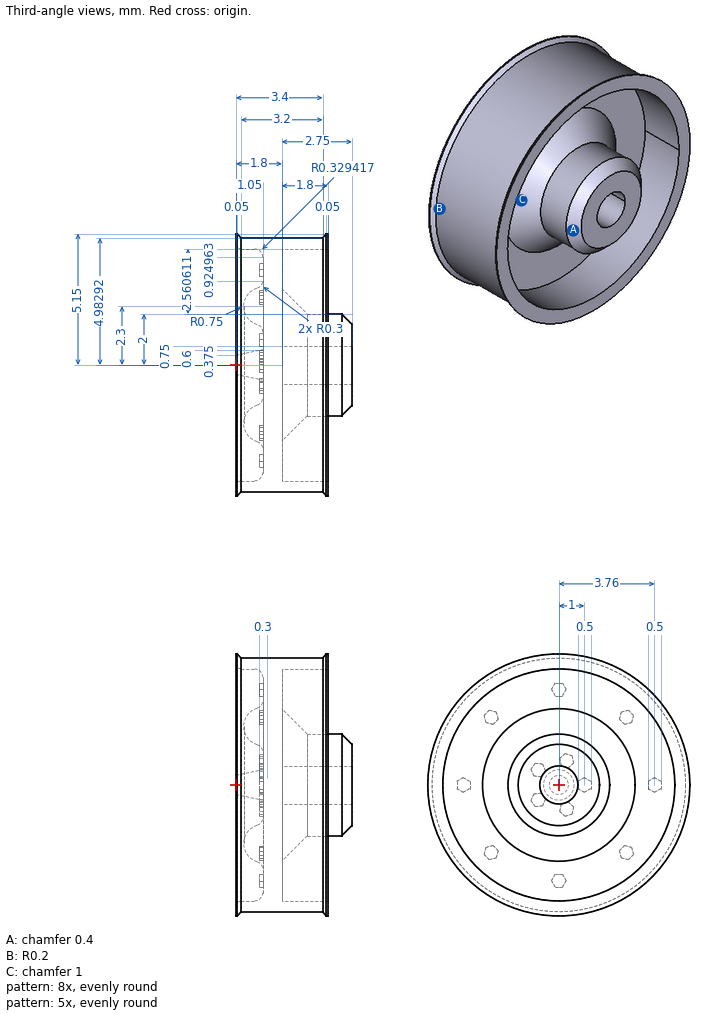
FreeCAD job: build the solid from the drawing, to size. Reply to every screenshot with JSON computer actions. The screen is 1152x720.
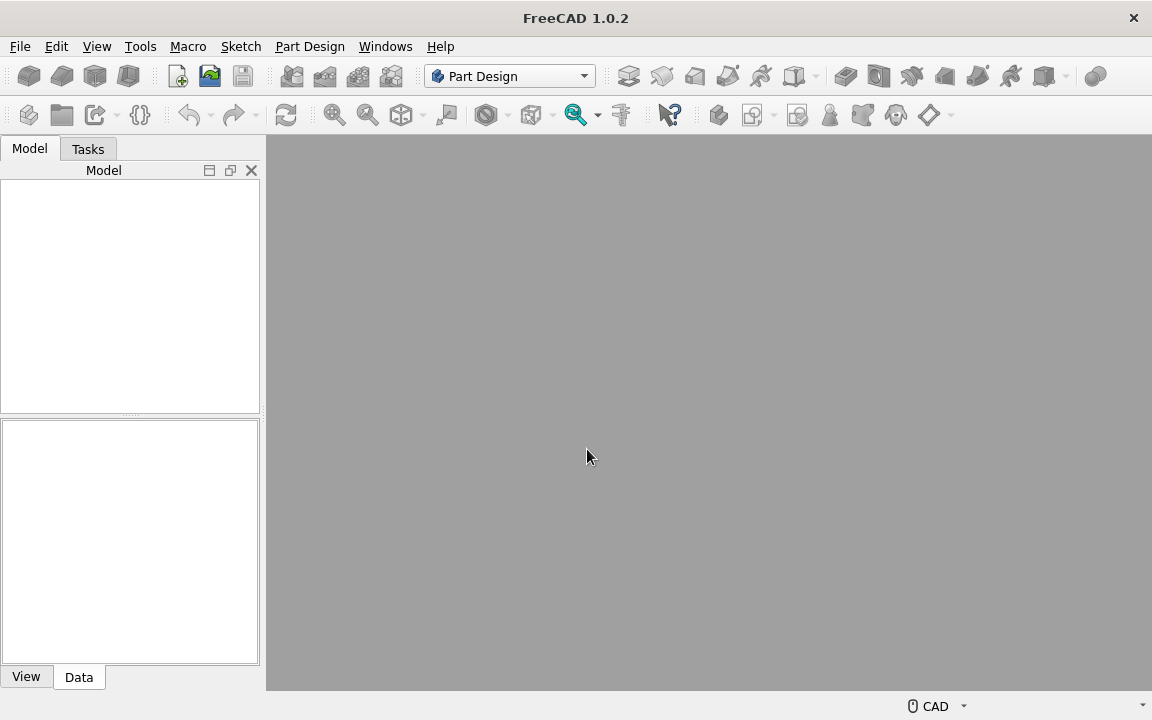
{"action": "left_click", "coordinate": [177, 76]}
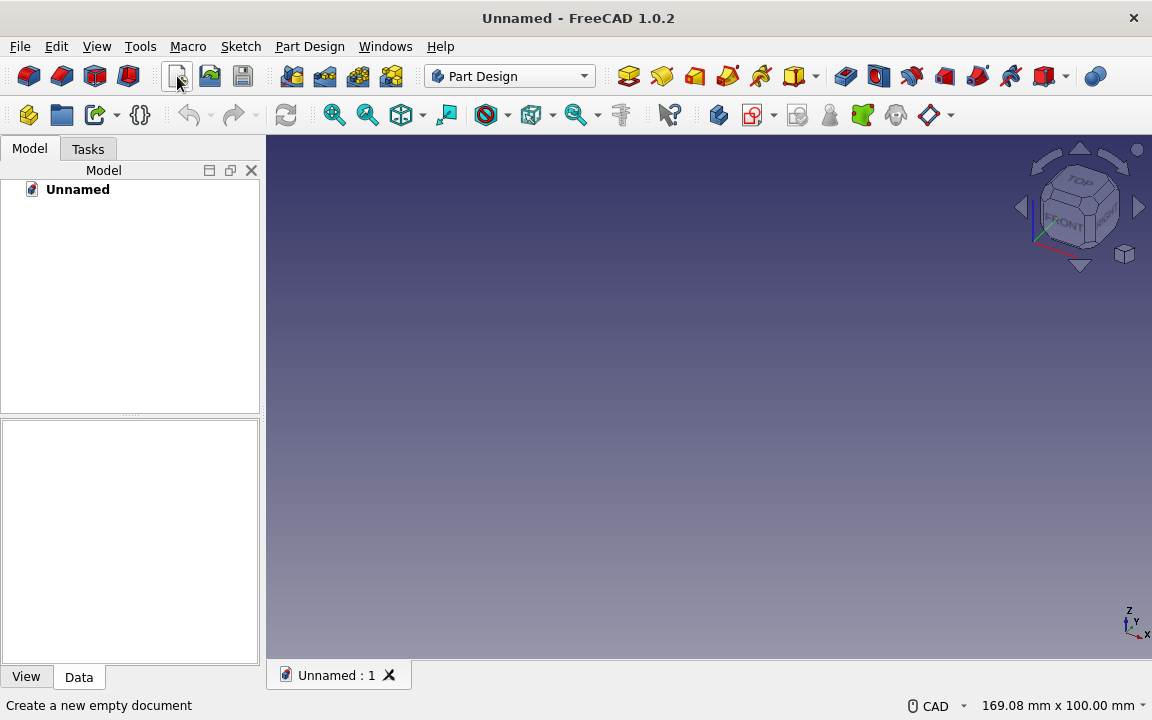
{"action": "left_click", "coordinate": [752, 116]}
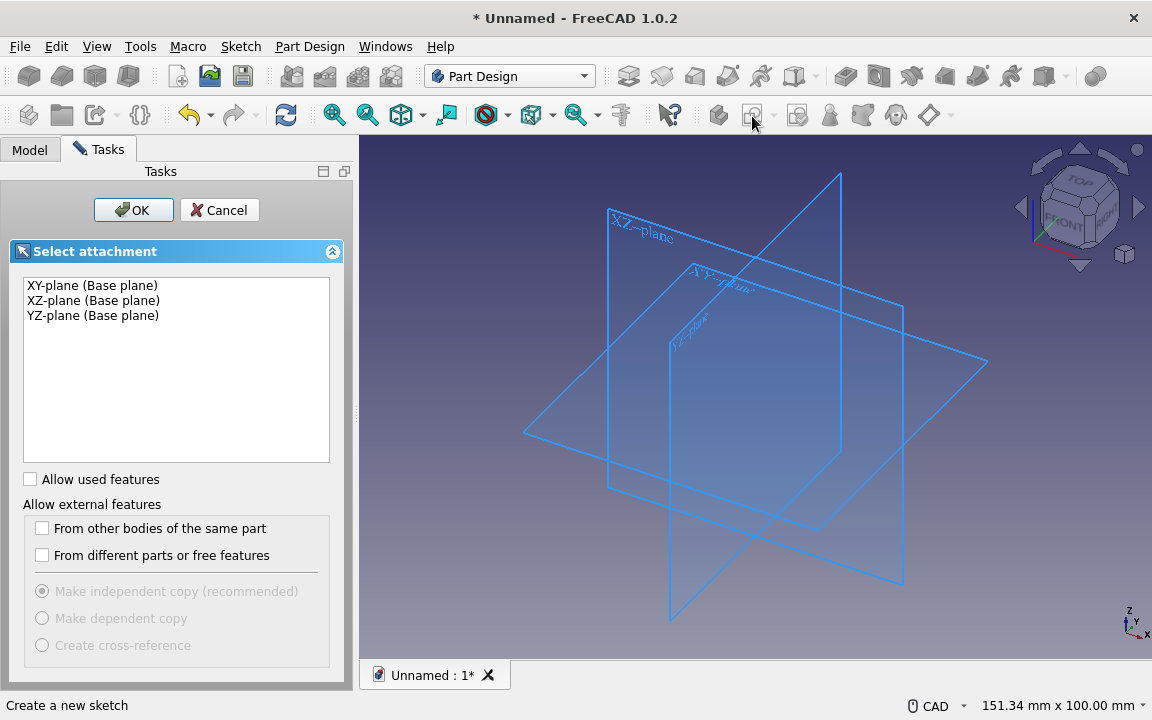
{"action": "left_click", "coordinate": [84, 286]}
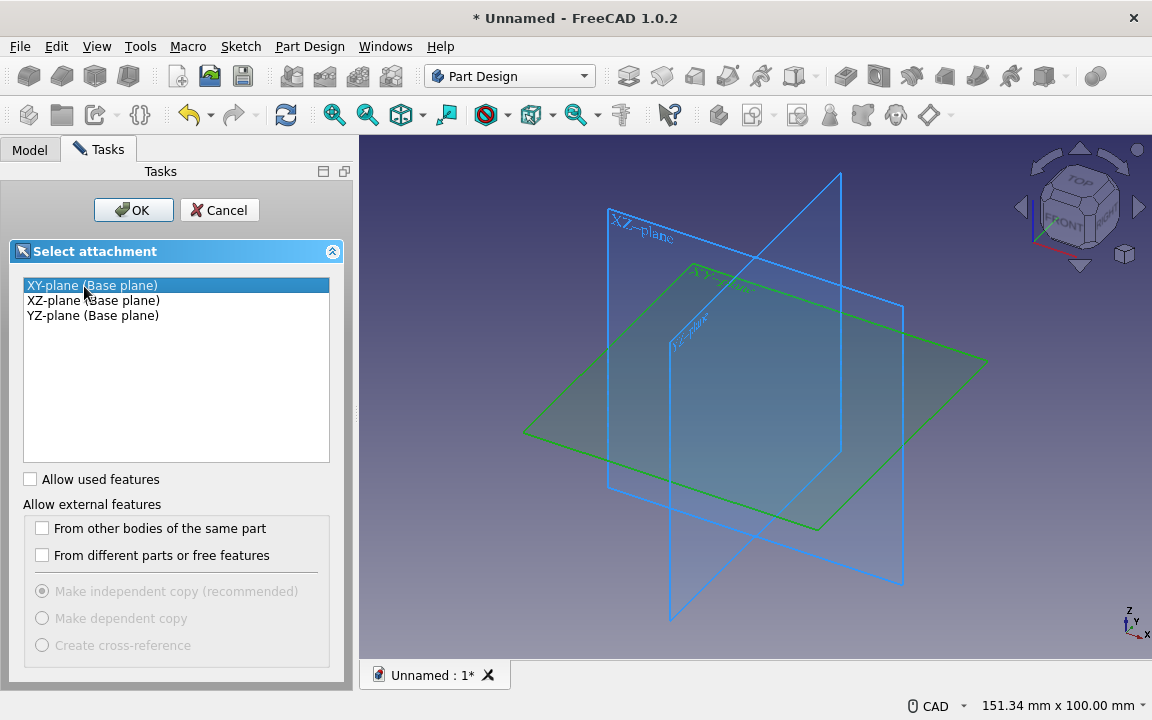
{"action": "left_click", "coordinate": [134, 210]}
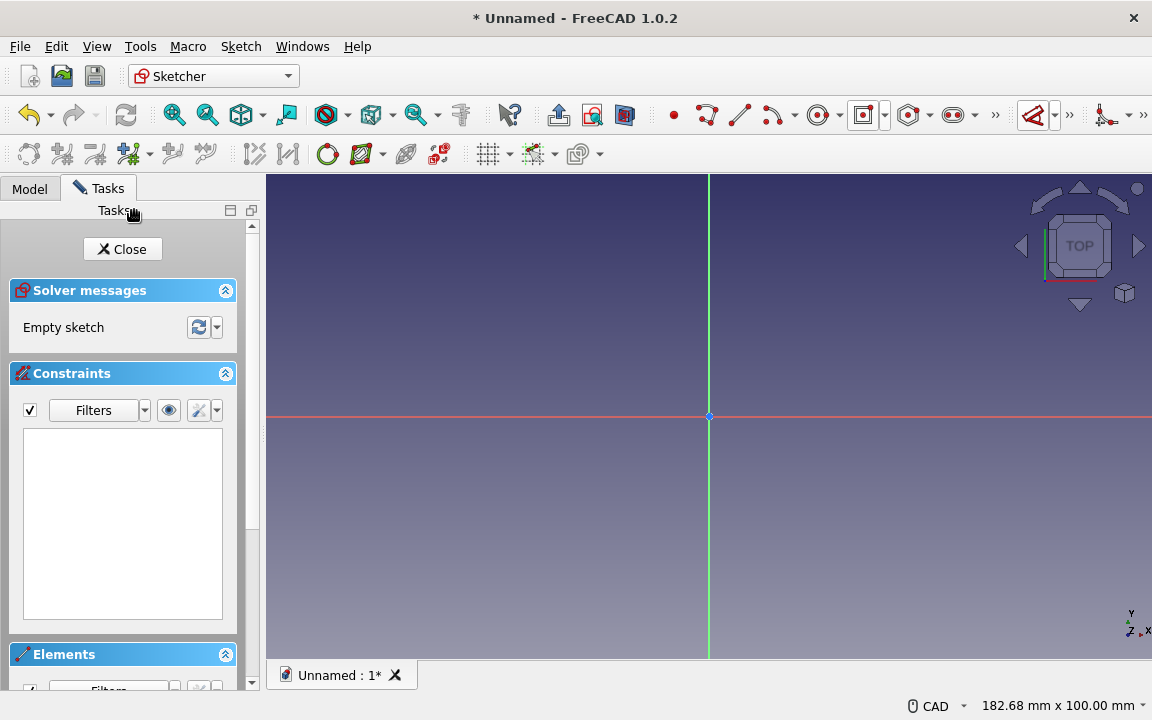
{"action": "scroll", "coordinate": [728, 403], "scroll_direction": "up", "scroll_amount": 12}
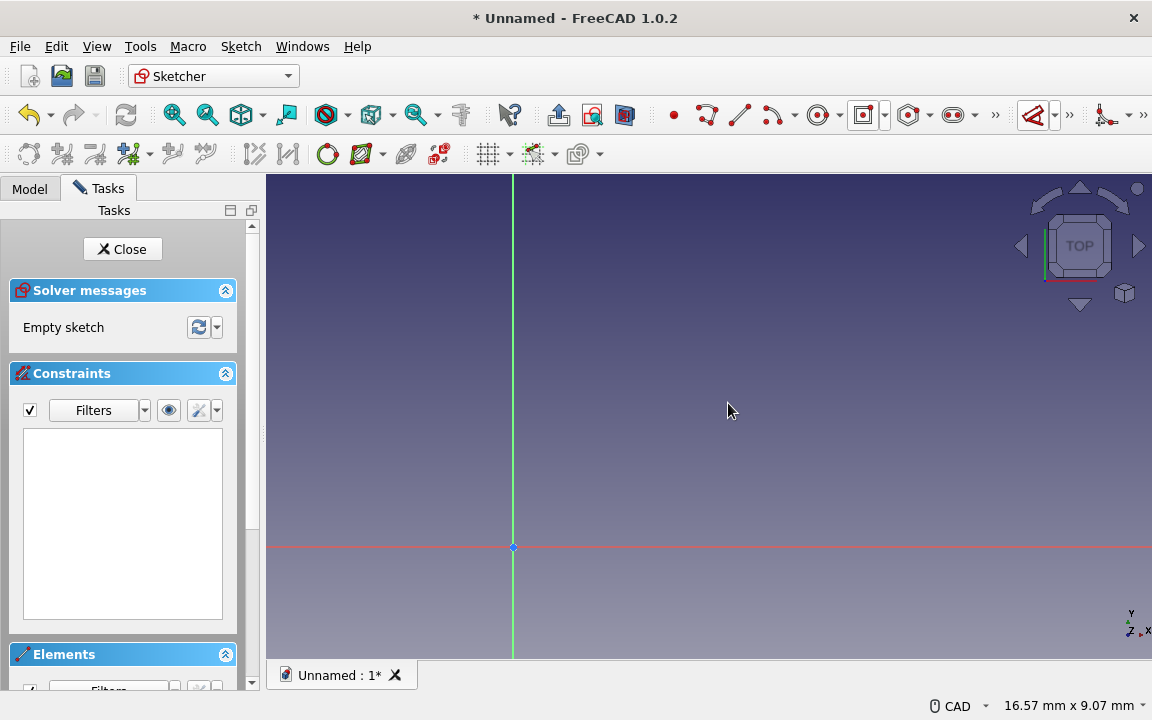
{"action": "left_click", "coordinate": [740, 116]}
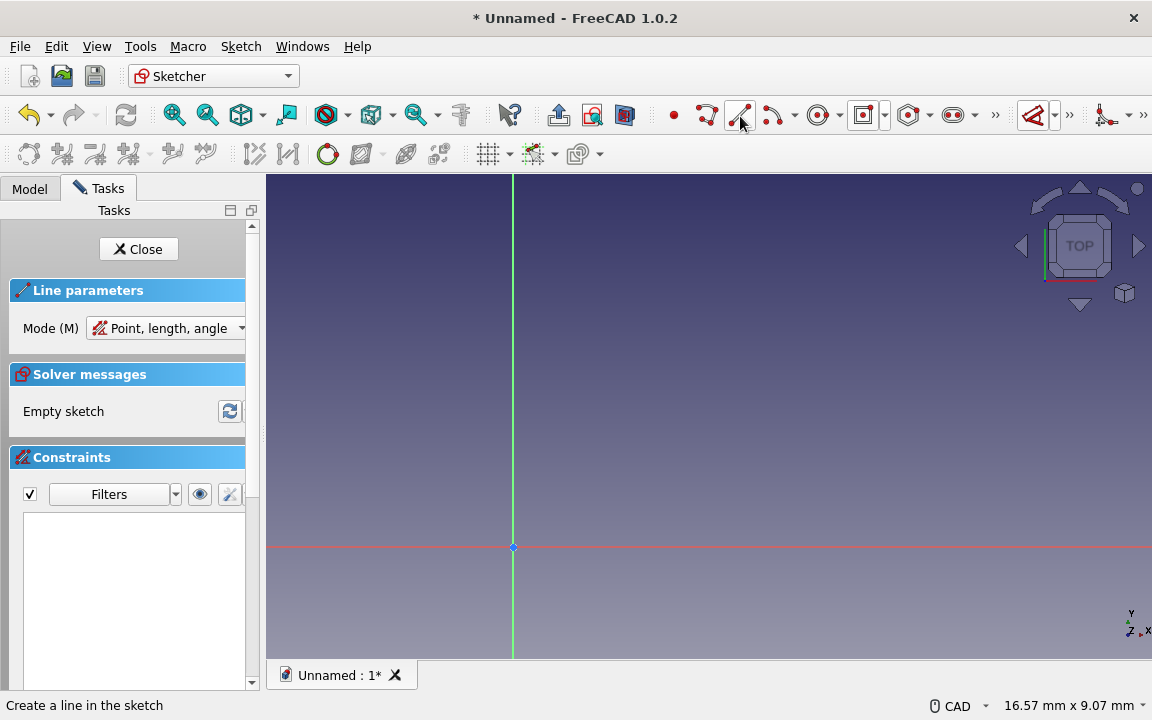
{"action": "left_click", "coordinate": [569, 321]}
{"action": "left_click", "coordinate": [569, 370]}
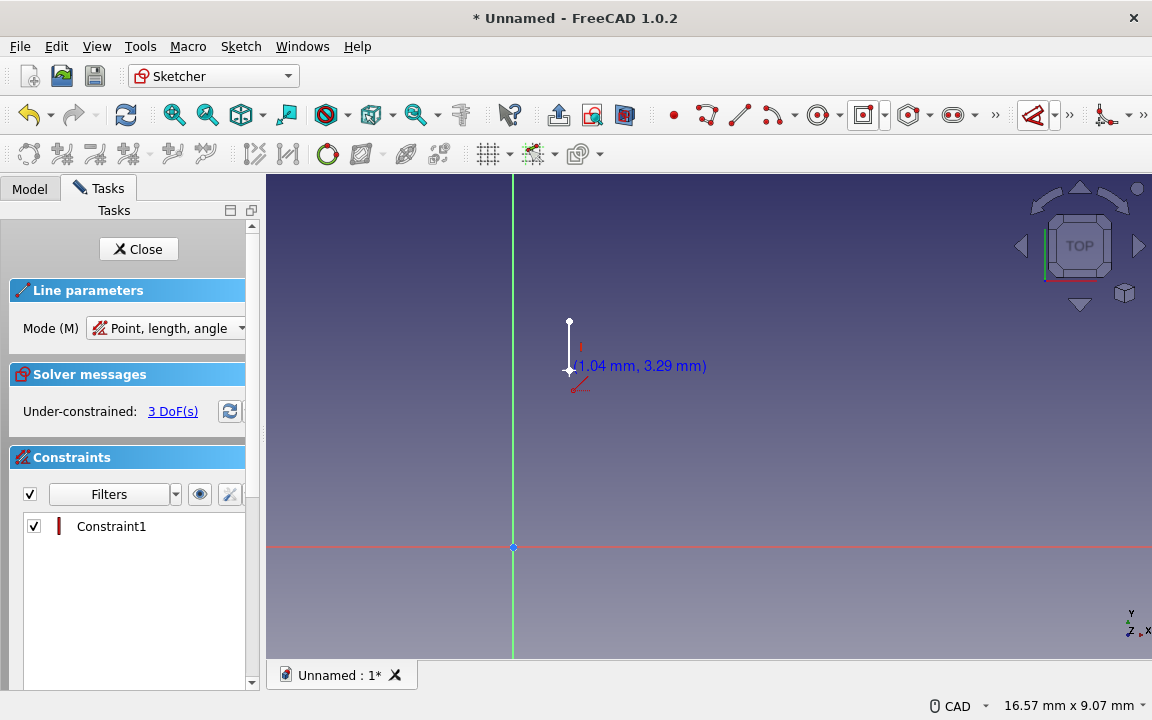
{"action": "left_click", "coordinate": [707, 116]}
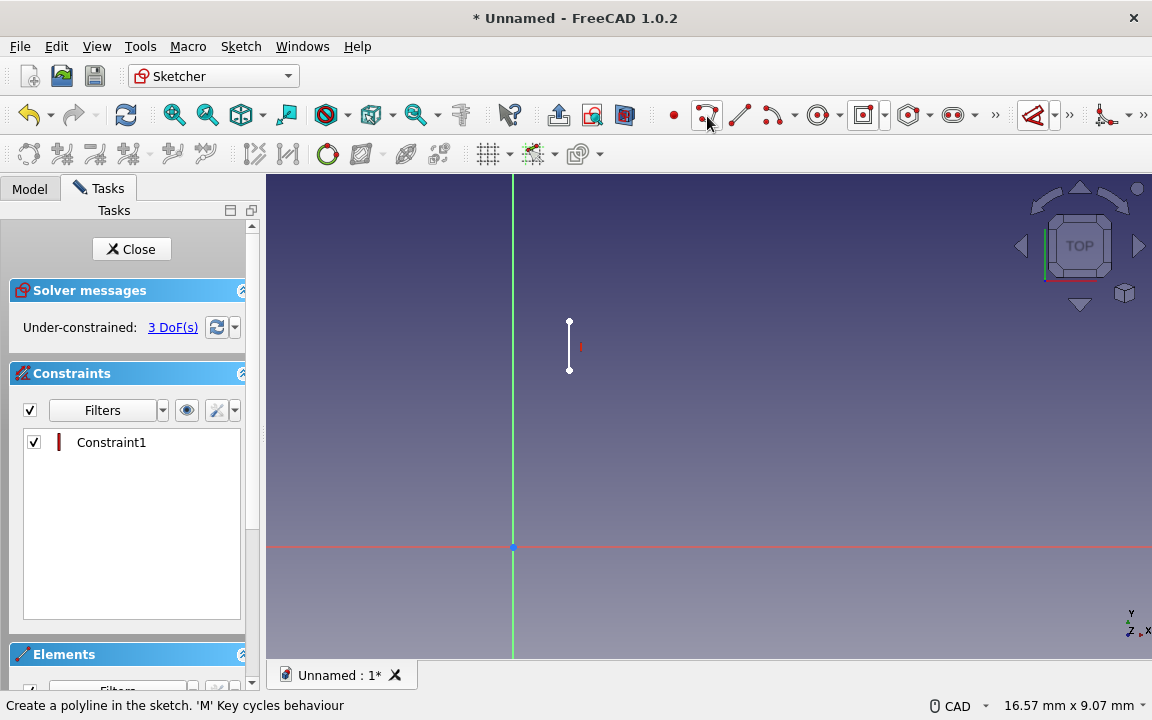
{"action": "left_click", "coordinate": [569, 478]}
{"action": "left_click", "coordinate": [569, 515]}
{"action": "left_click", "coordinate": [513, 527]}
{"action": "left_click", "coordinate": [513, 547]}
{"action": "left_click", "coordinate": [610, 538]}
{"action": "left_click", "coordinate": [610, 507]}
{"action": "left_click", "coordinate": [757, 507]}
{"action": "left_click", "coordinate": [757, 440]}
{"action": "left_click", "coordinate": [610, 440]}
{"action": "left_click", "coordinate": [610, 303]}
{"action": "left_click", "coordinate": [706, 303]}
{"action": "left_click", "coordinate": [706, 272]}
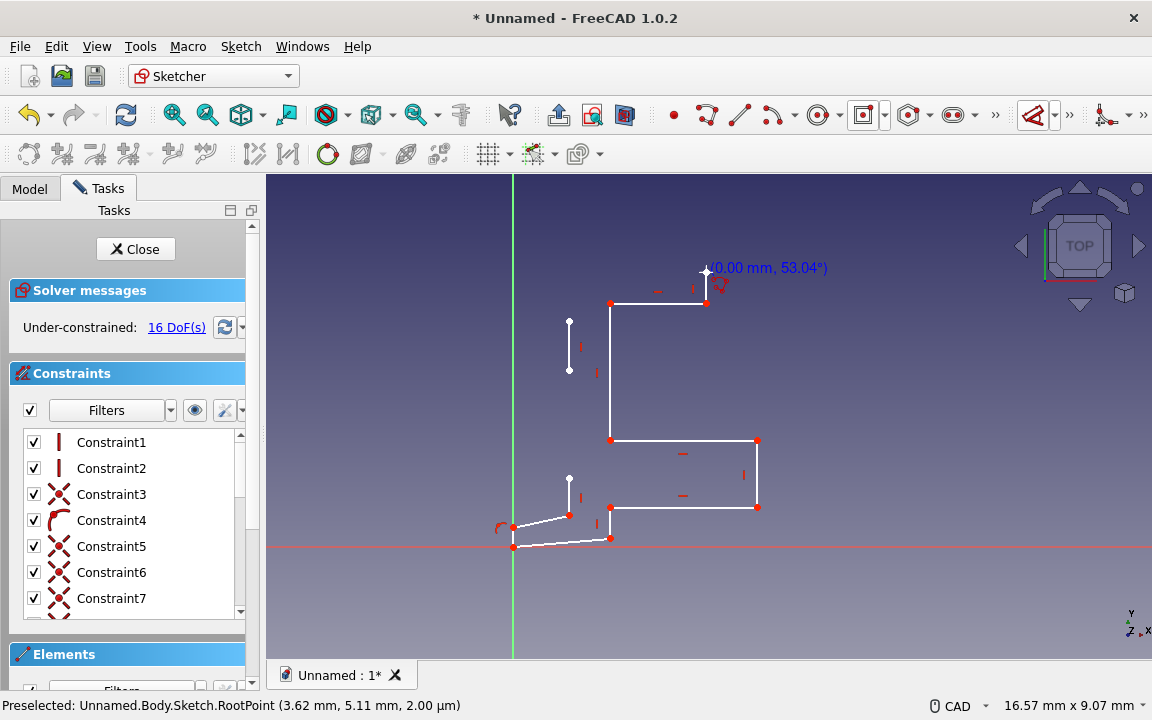
{"action": "scroll", "coordinate": [703, 272], "scroll_direction": "up", "scroll_amount": 9}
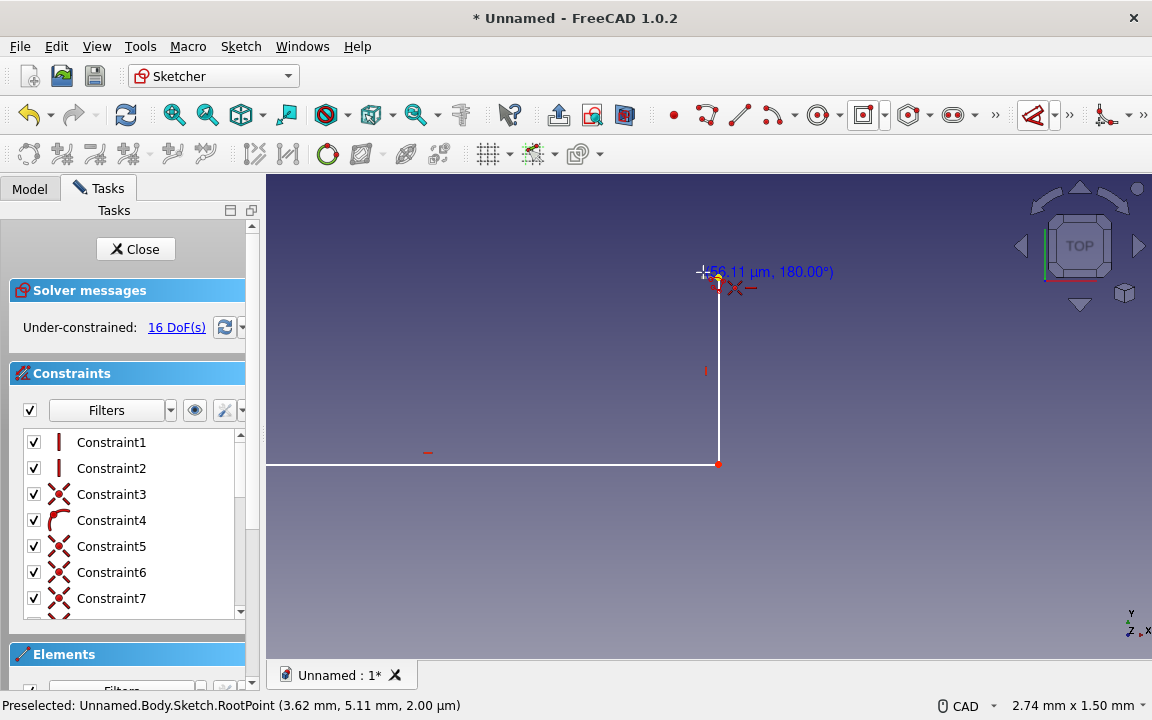
{"action": "left_click", "coordinate": [701, 271]}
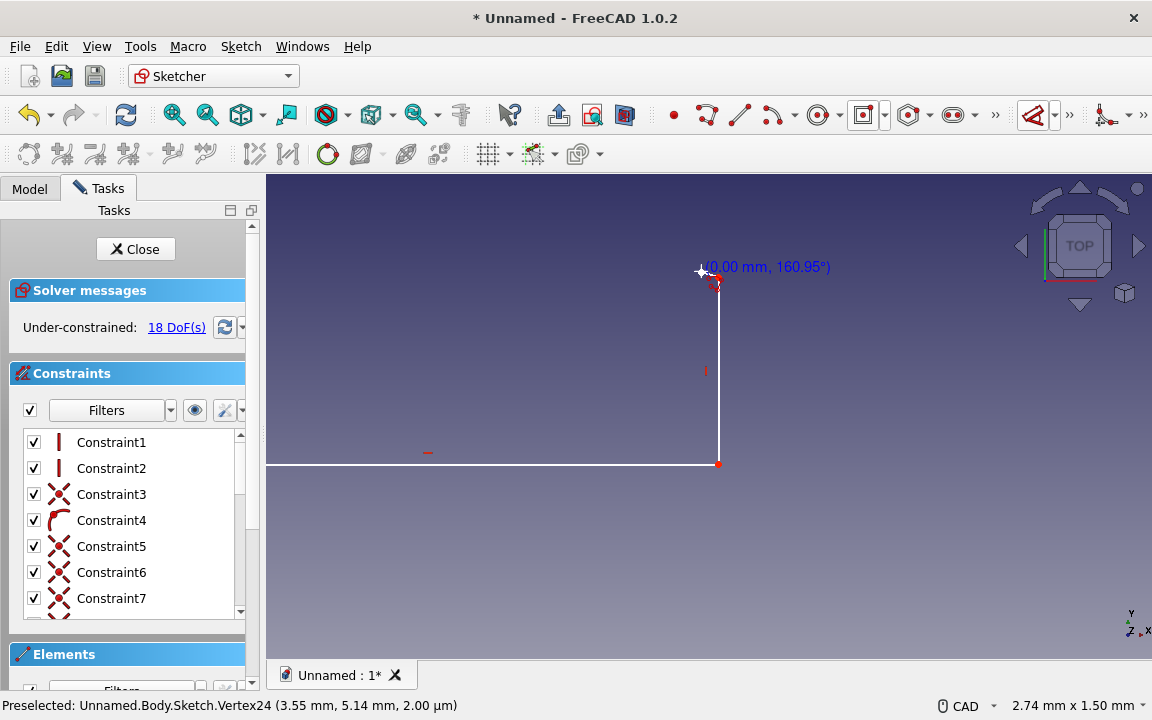
{"action": "scroll", "coordinate": [710, 281], "scroll_direction": "down", "scroll_amount": 9}